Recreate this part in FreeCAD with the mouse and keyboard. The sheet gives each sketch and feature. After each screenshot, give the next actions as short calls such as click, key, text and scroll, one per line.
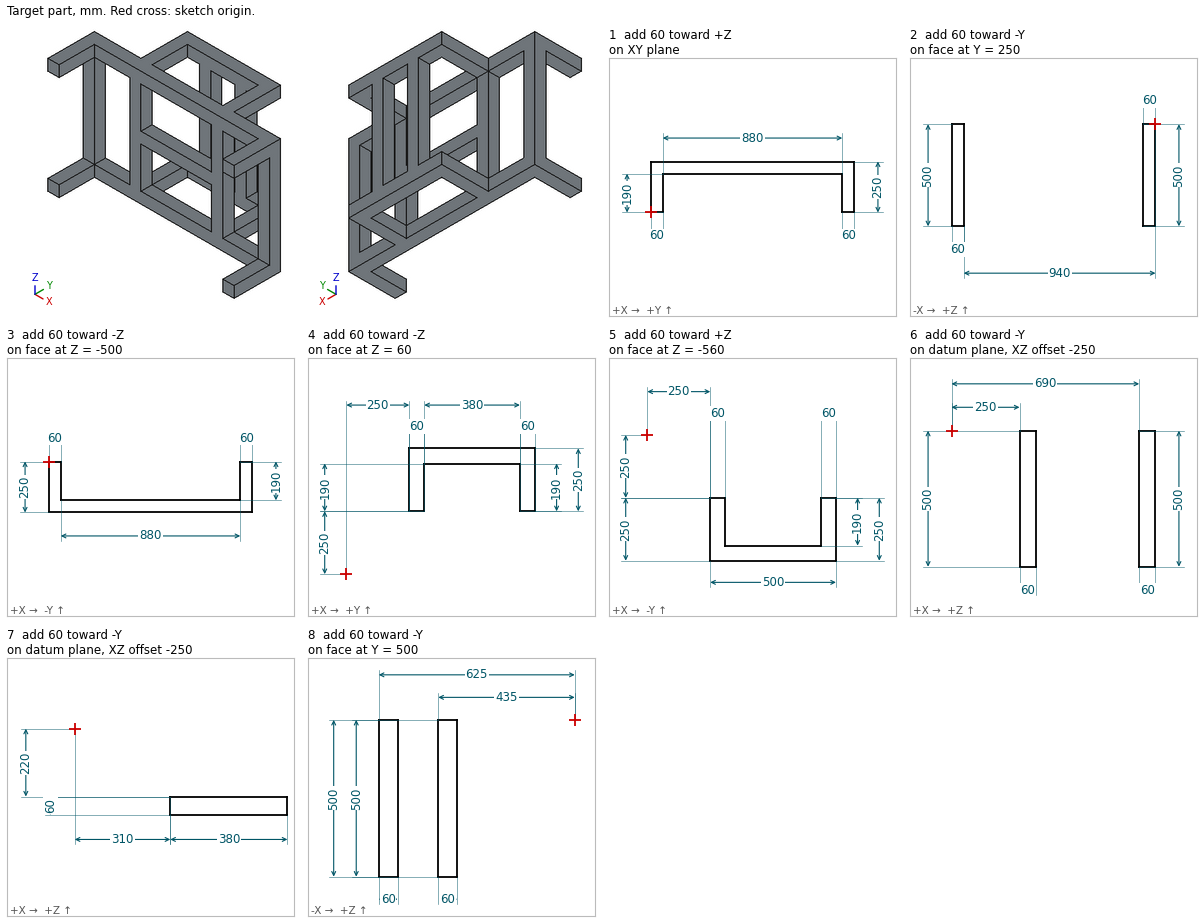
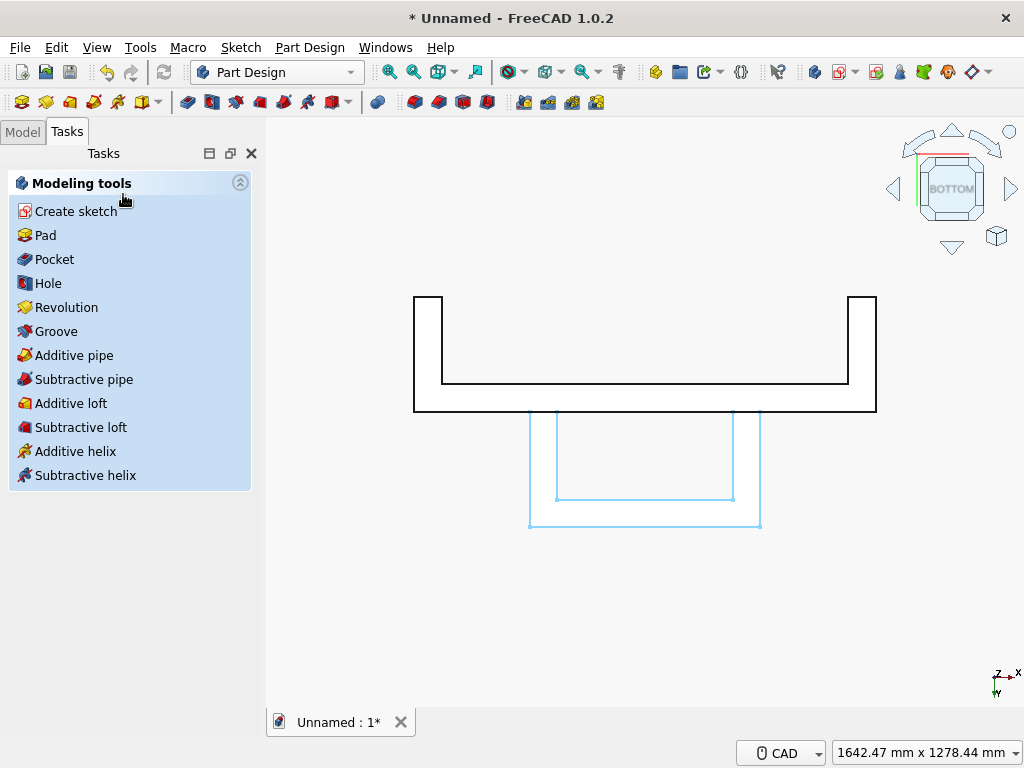
click(22, 102)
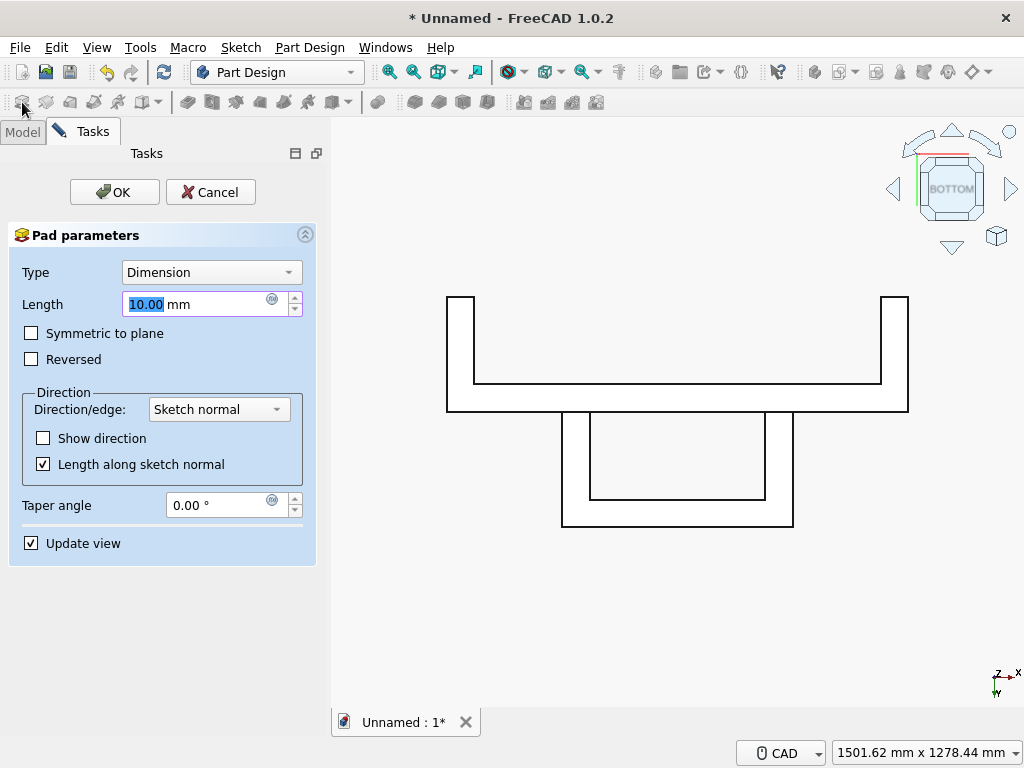
text(60)
key(Tab)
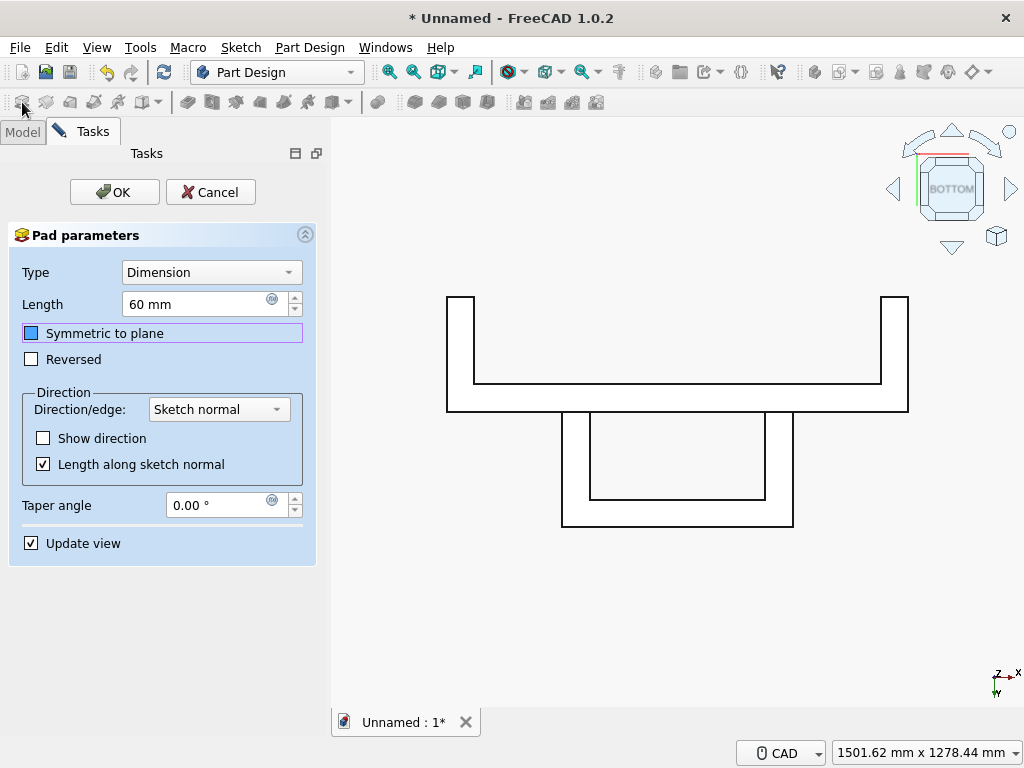
click(30, 359)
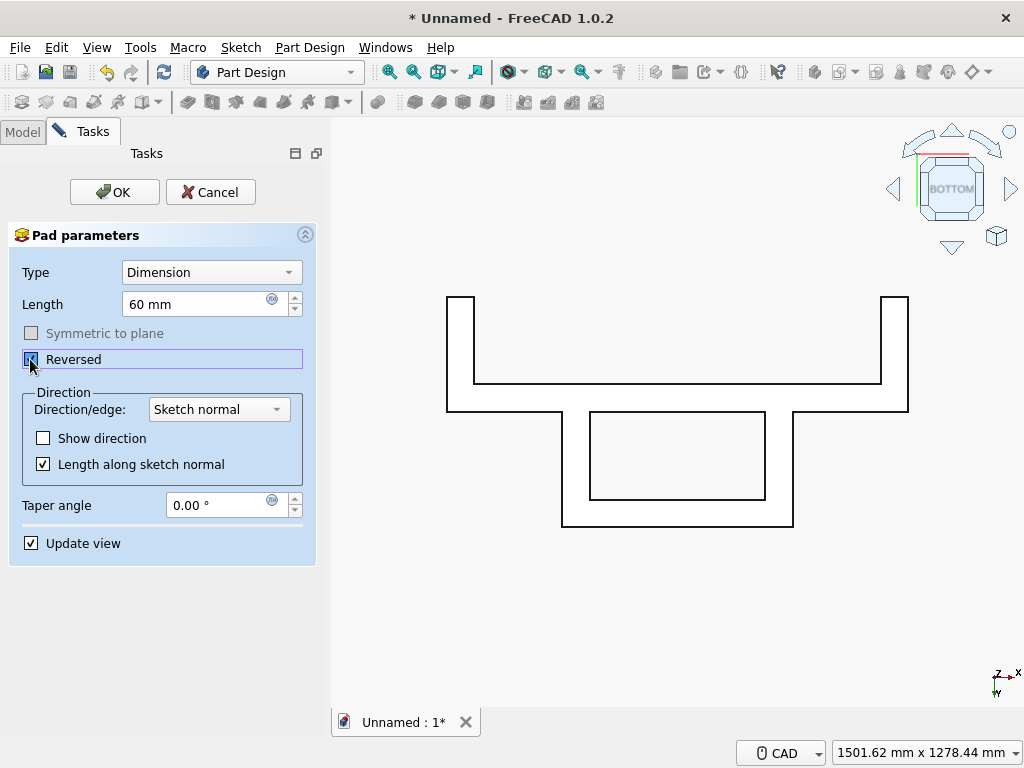
click(115, 192)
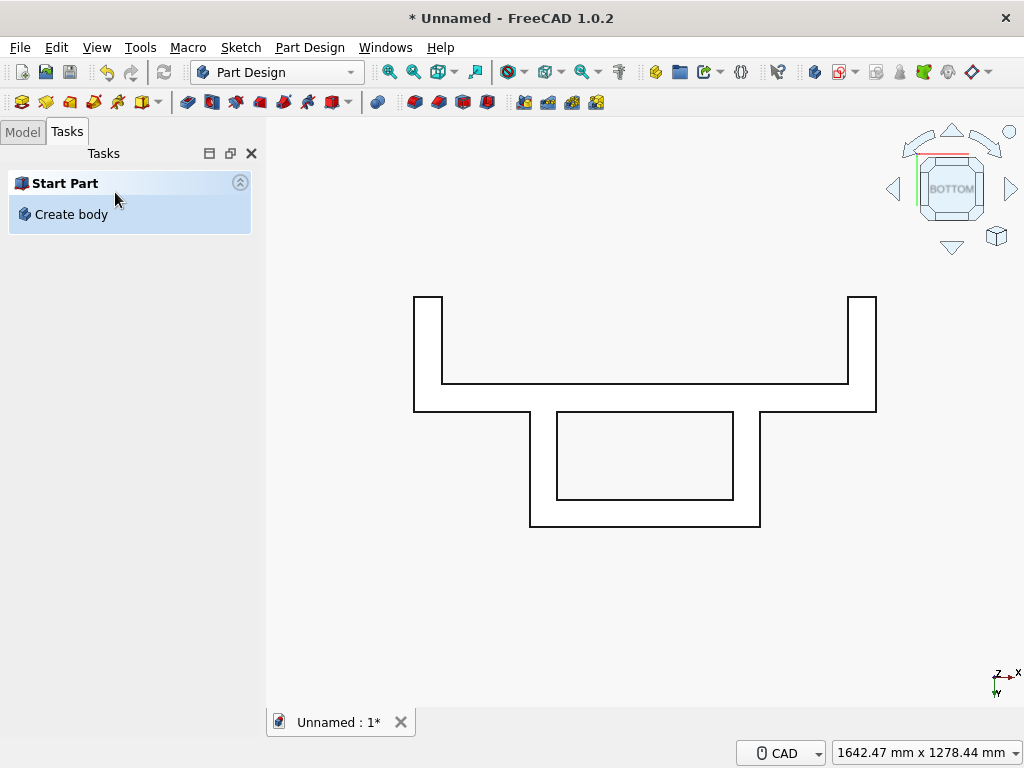
key(4)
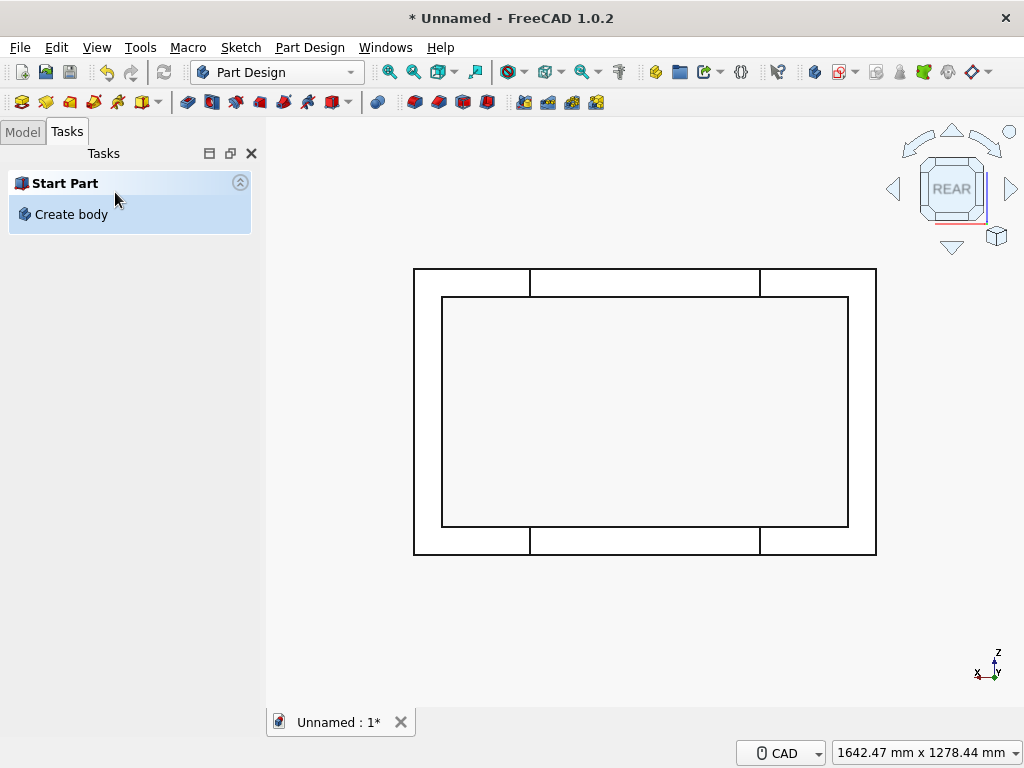
key(2)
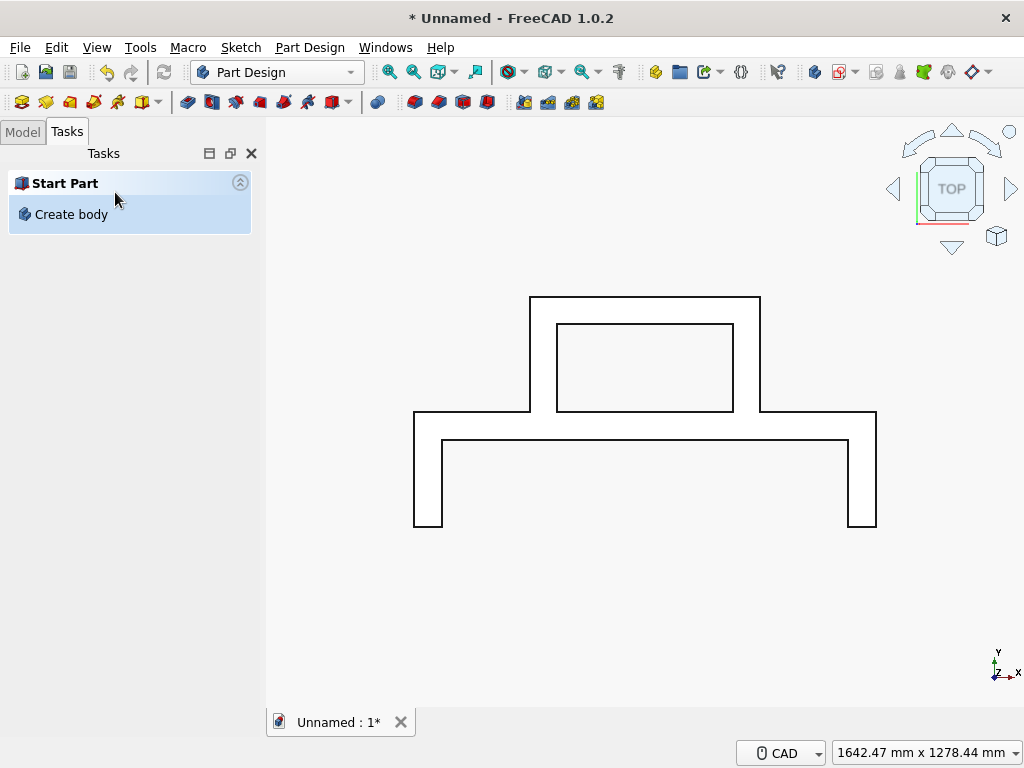
key(3)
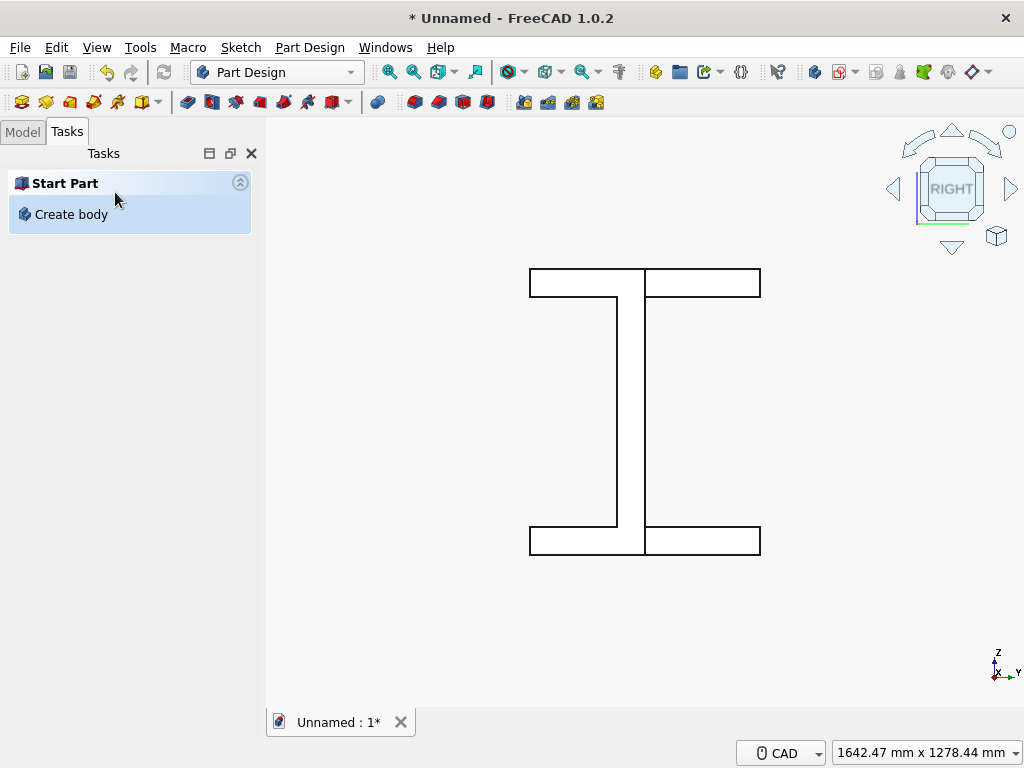
click(23, 131)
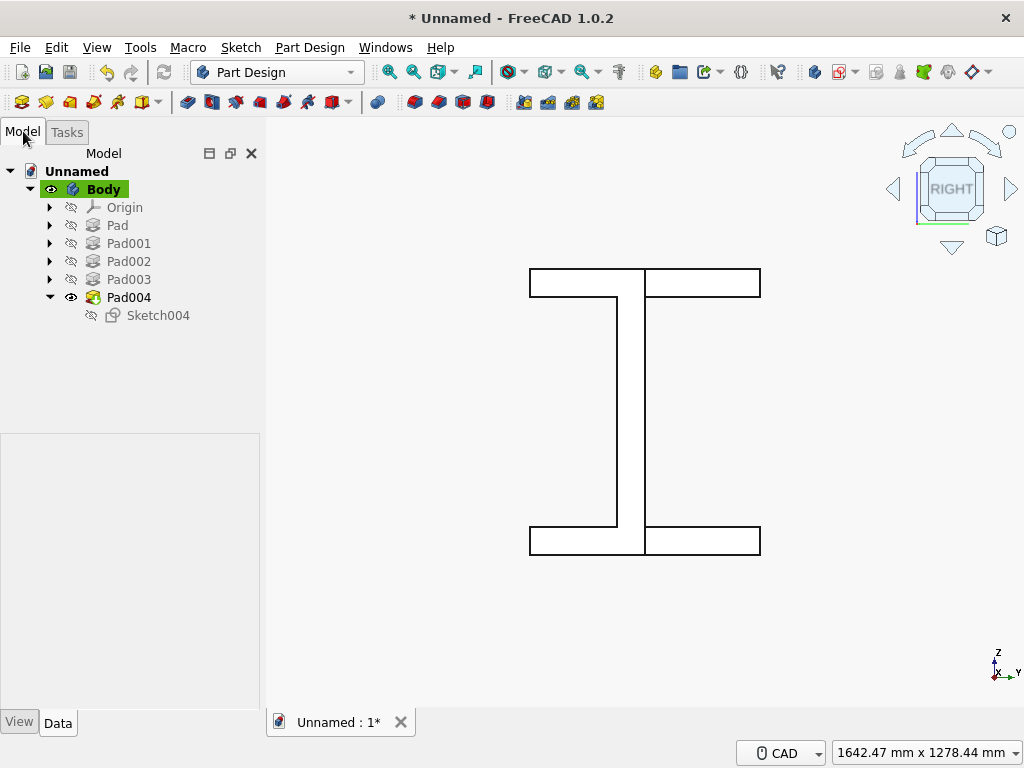
click(50, 207)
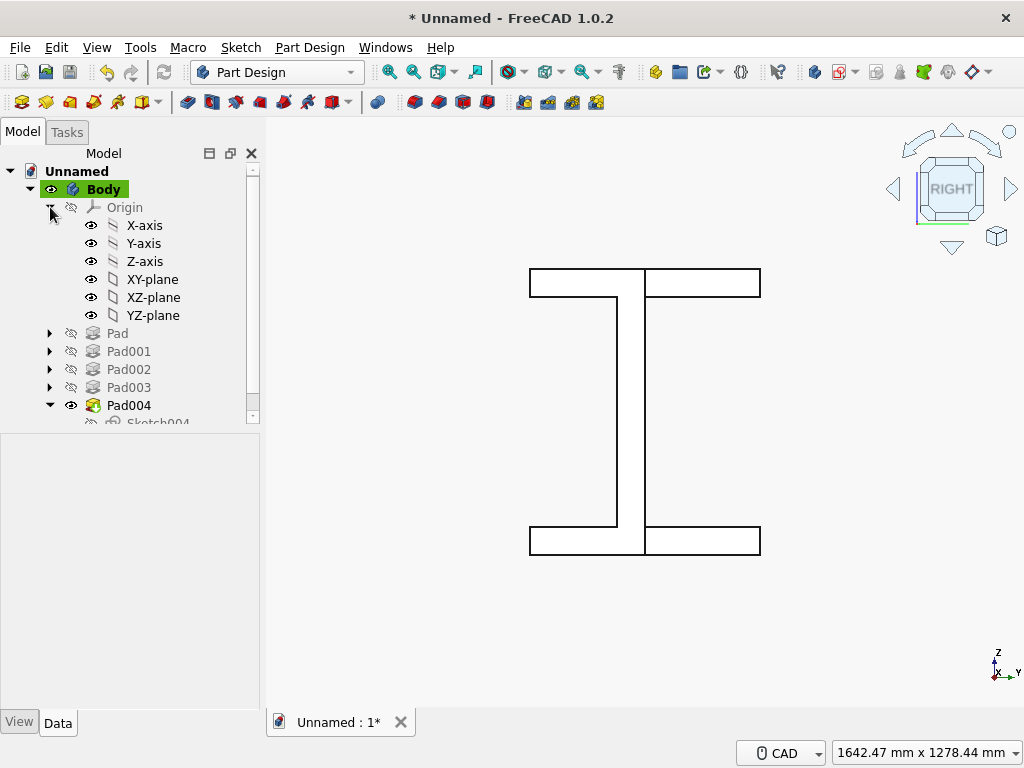
click(136, 297)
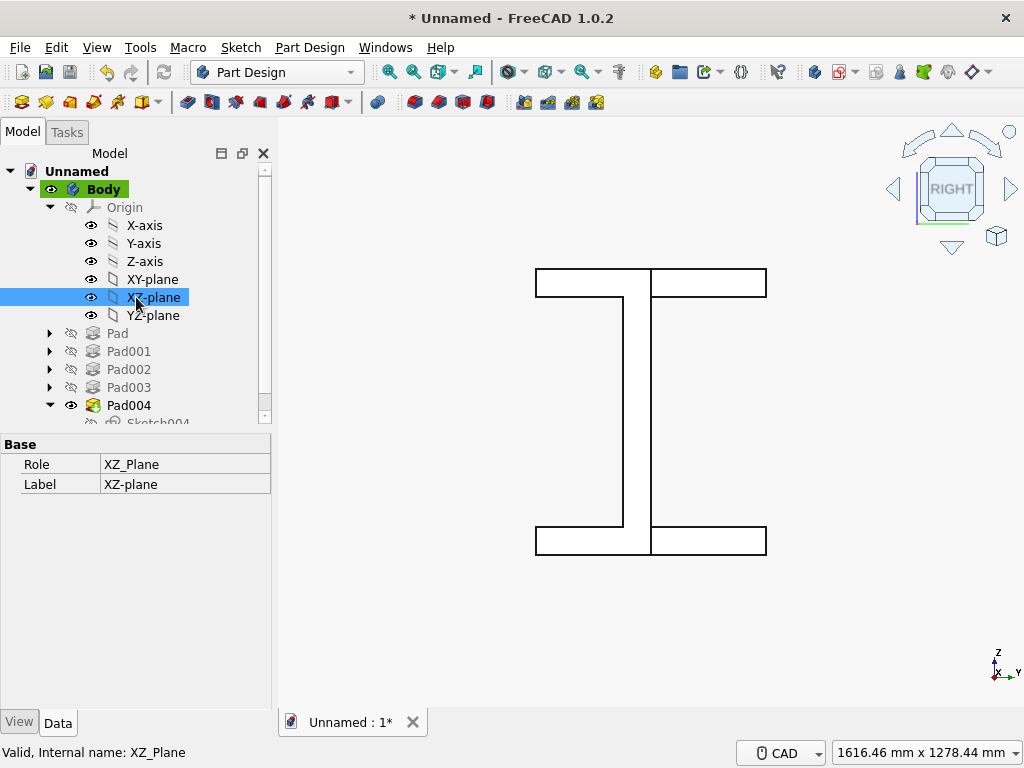
click(972, 72)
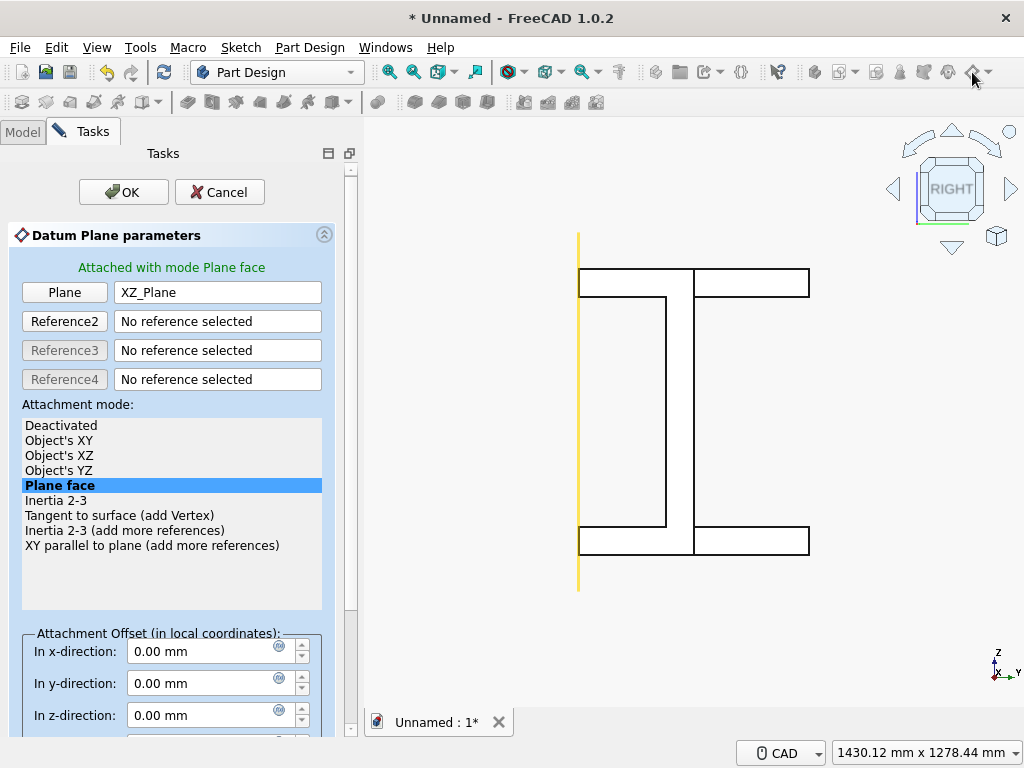
triple_click(210, 715)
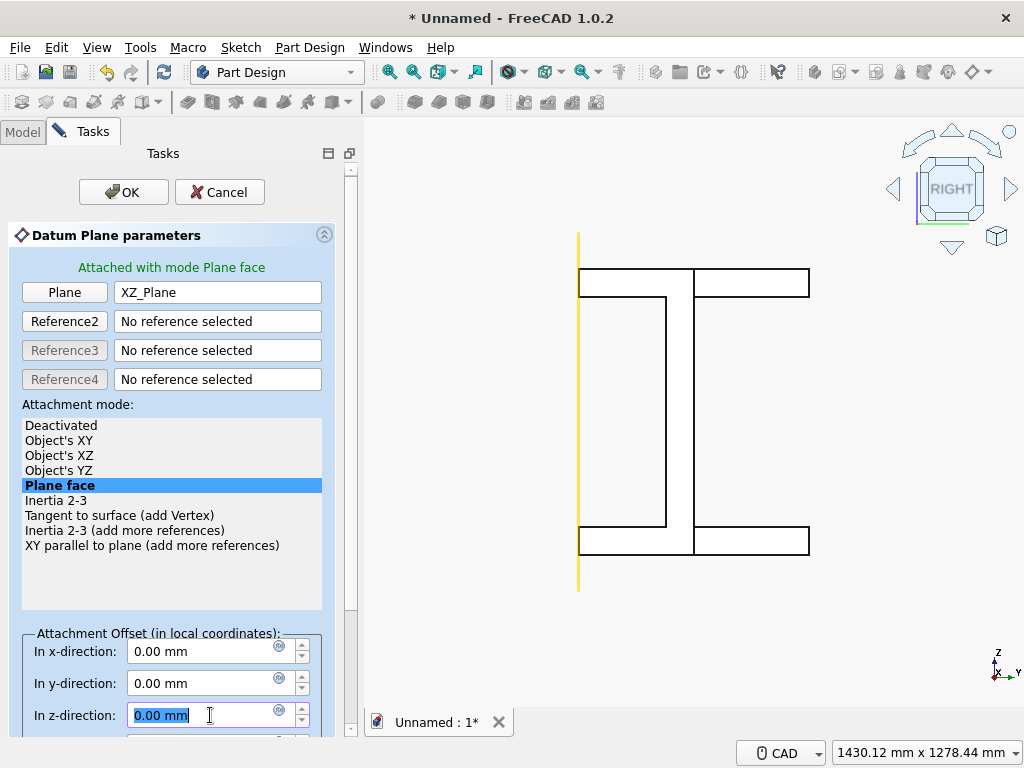
text(-250)
key(Tab)